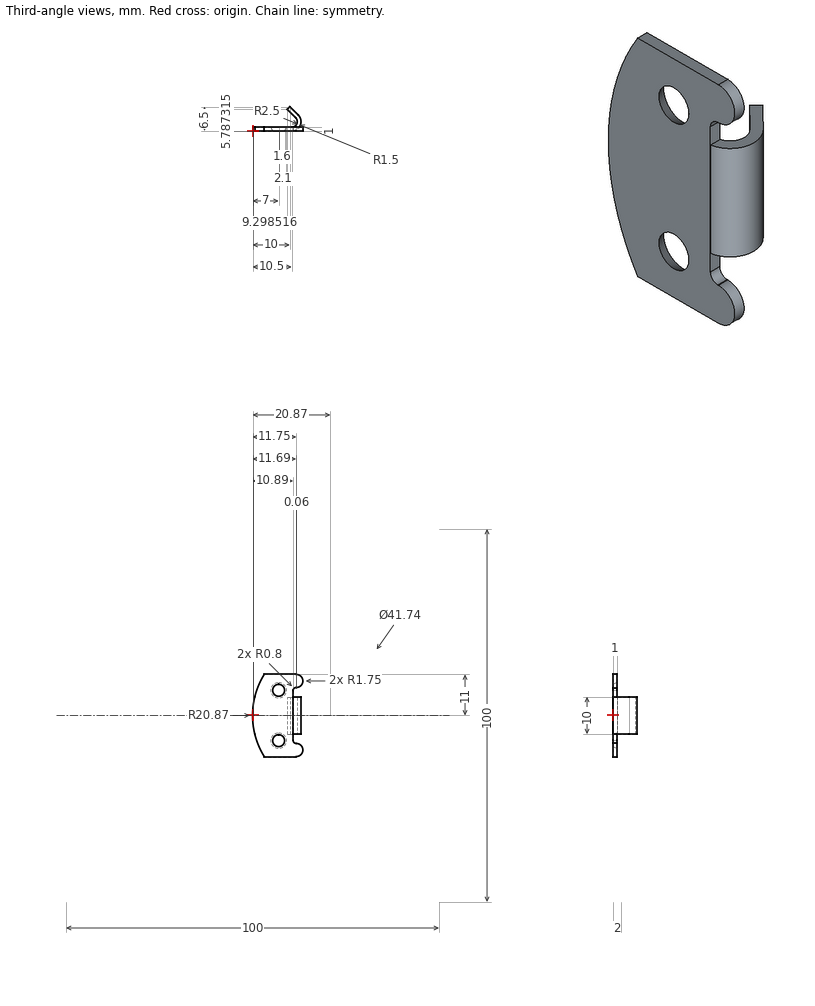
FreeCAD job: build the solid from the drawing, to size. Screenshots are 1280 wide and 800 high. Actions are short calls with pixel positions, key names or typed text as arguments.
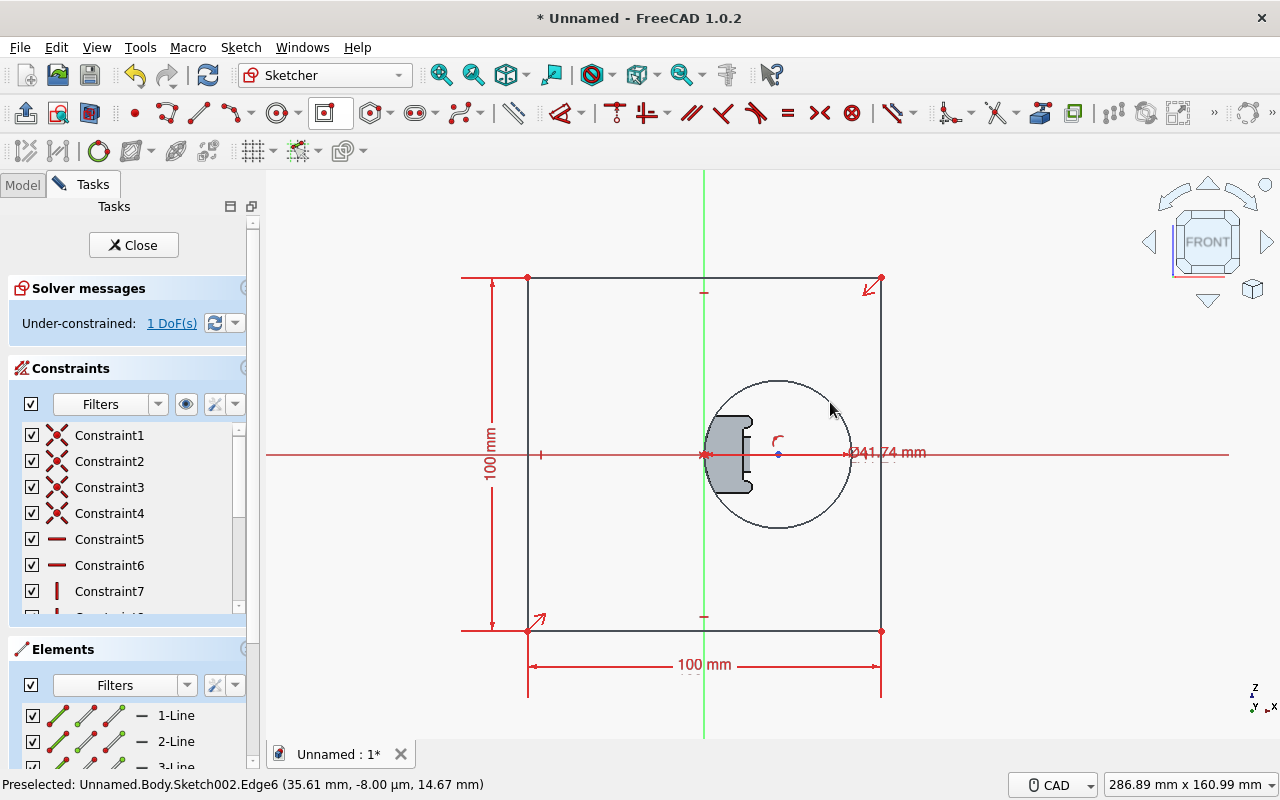
click(560, 114)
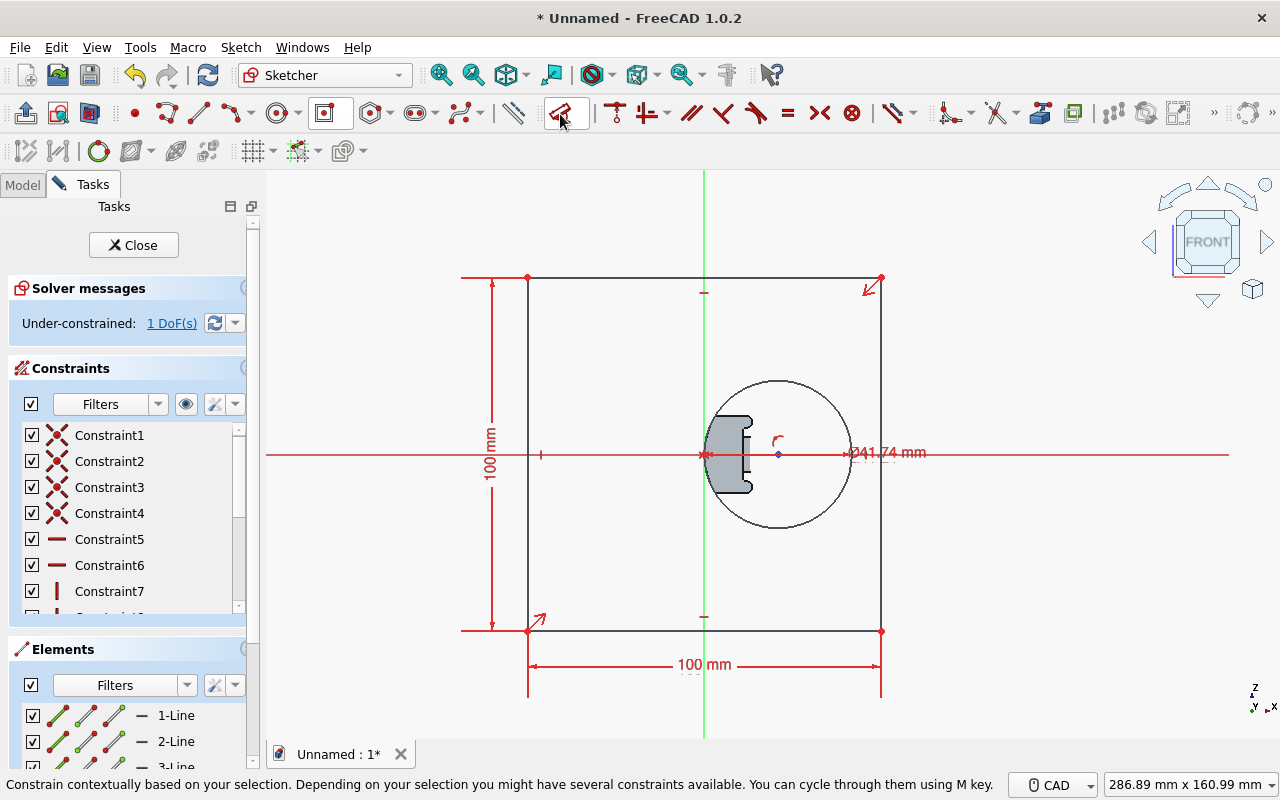
click(778, 455)
click(741, 489)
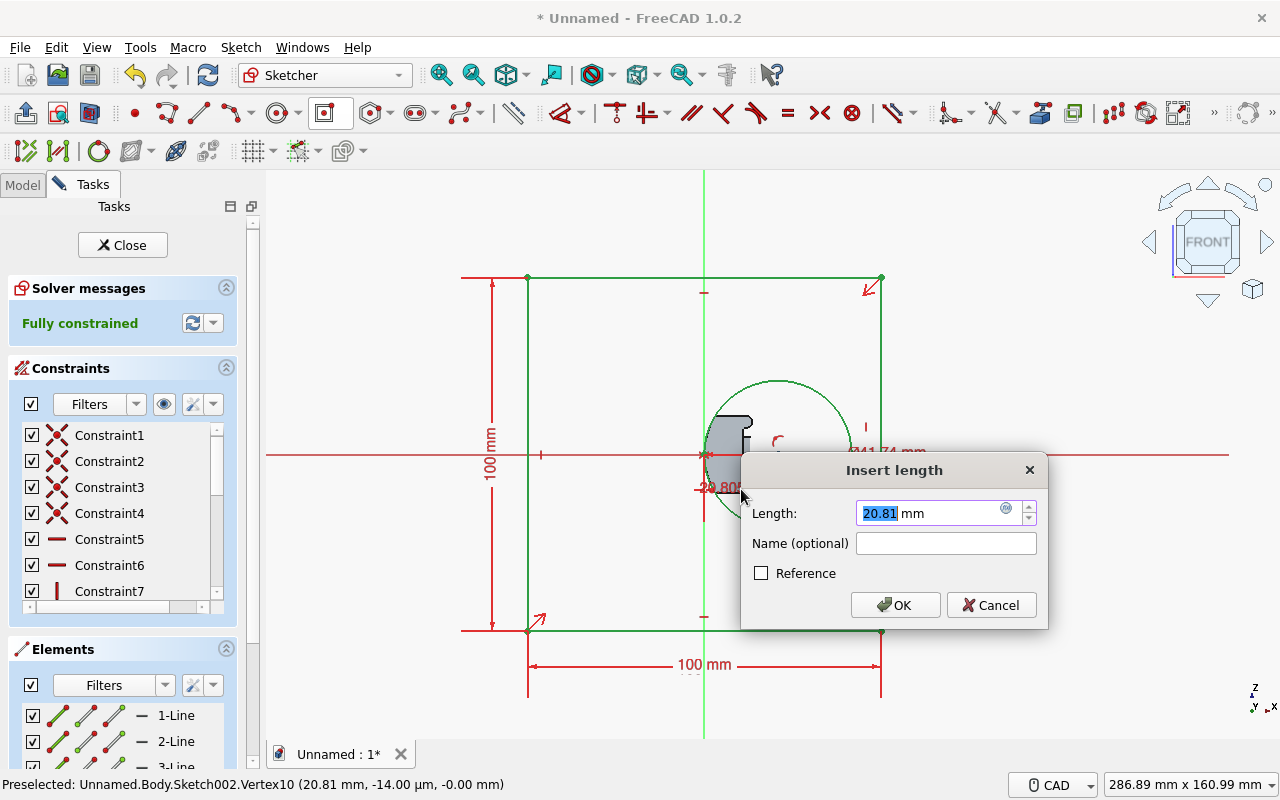
text(20.87)
key(Return)
key(Escape)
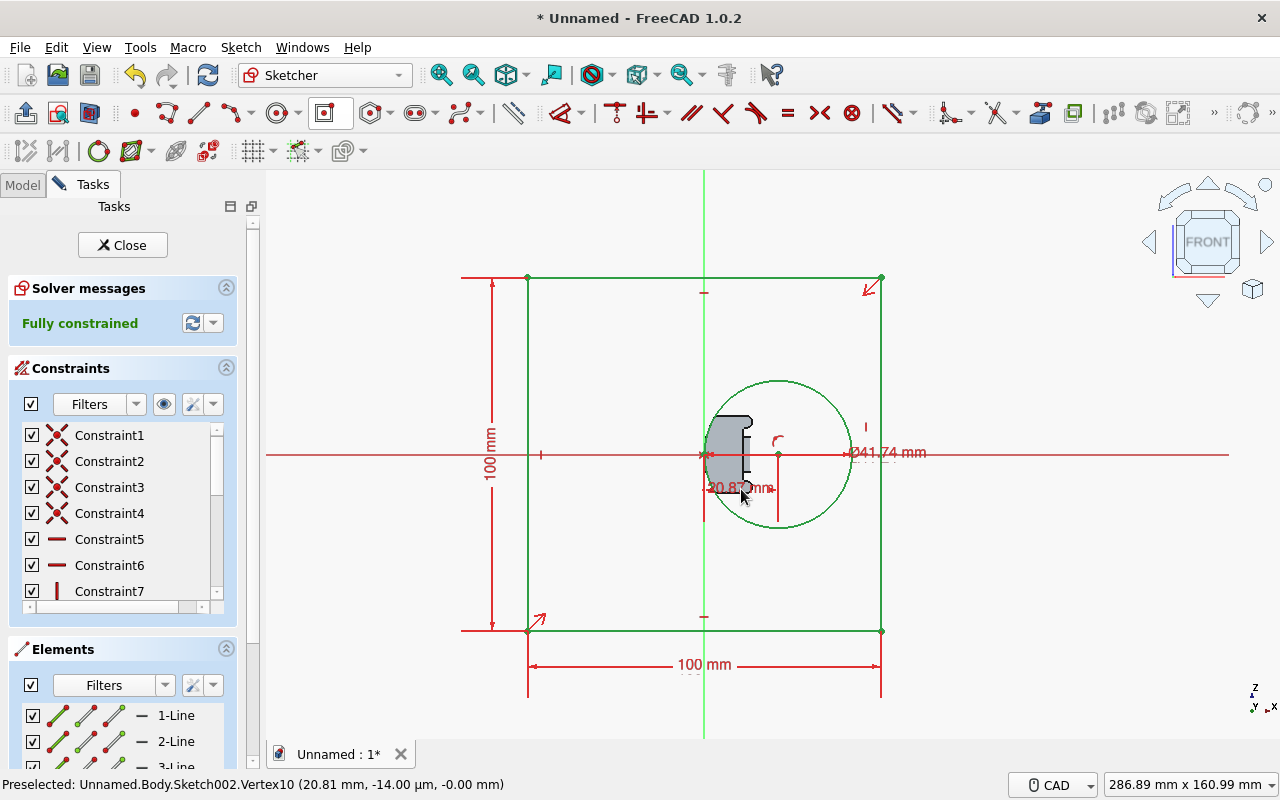
click(123, 245)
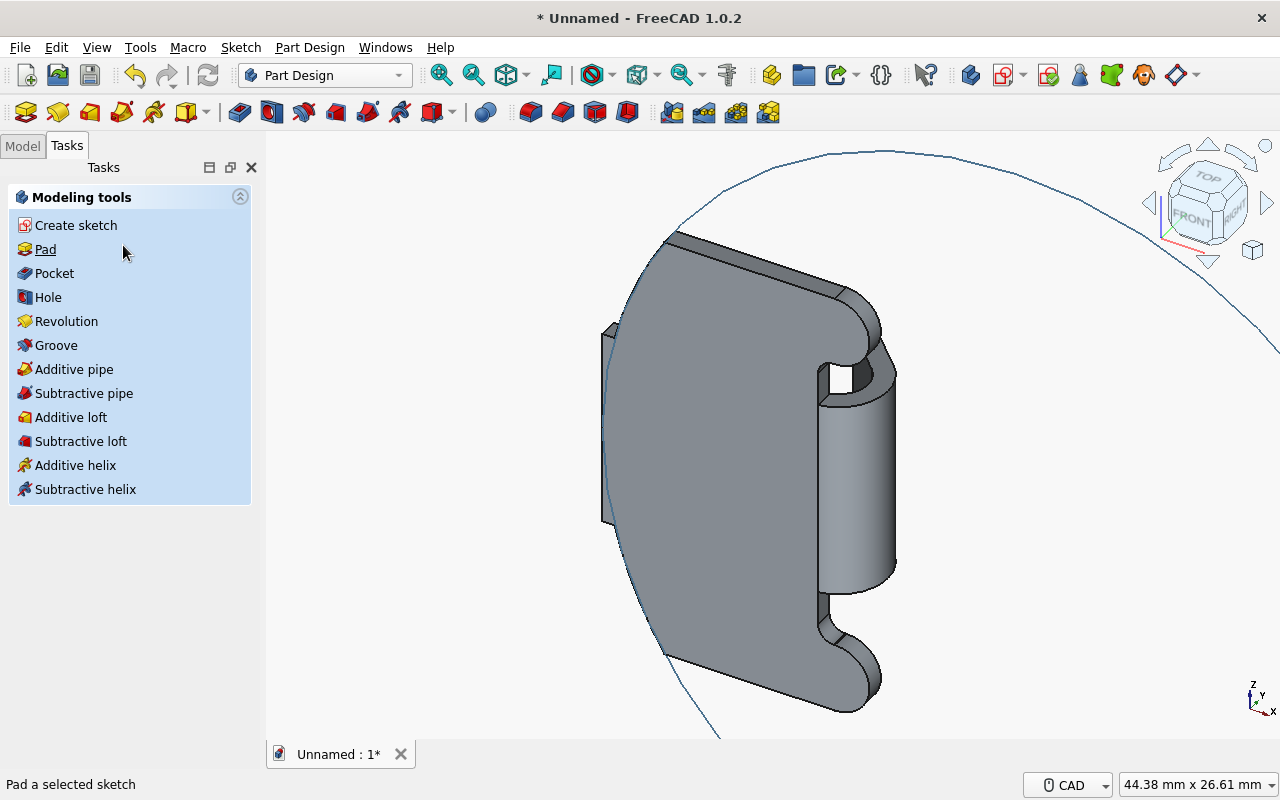
click(240, 112)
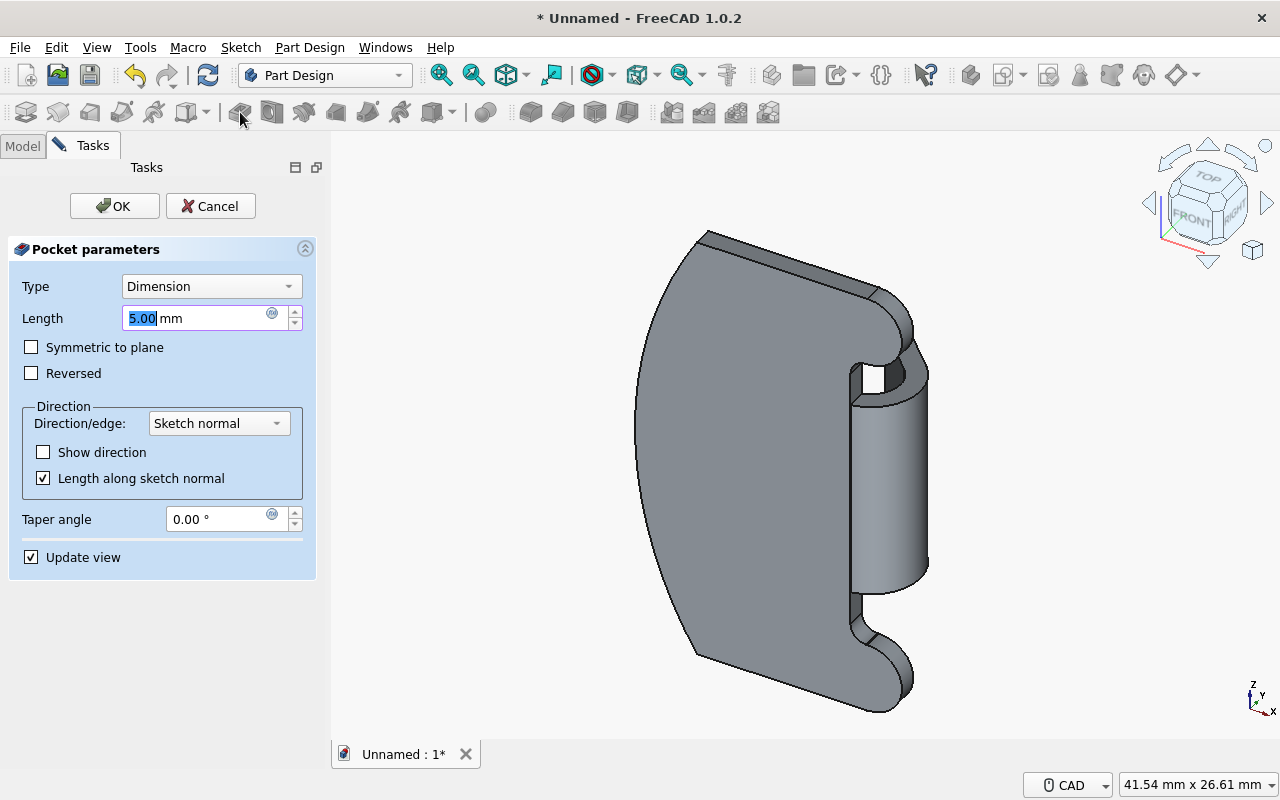
text(2)
key(Tab)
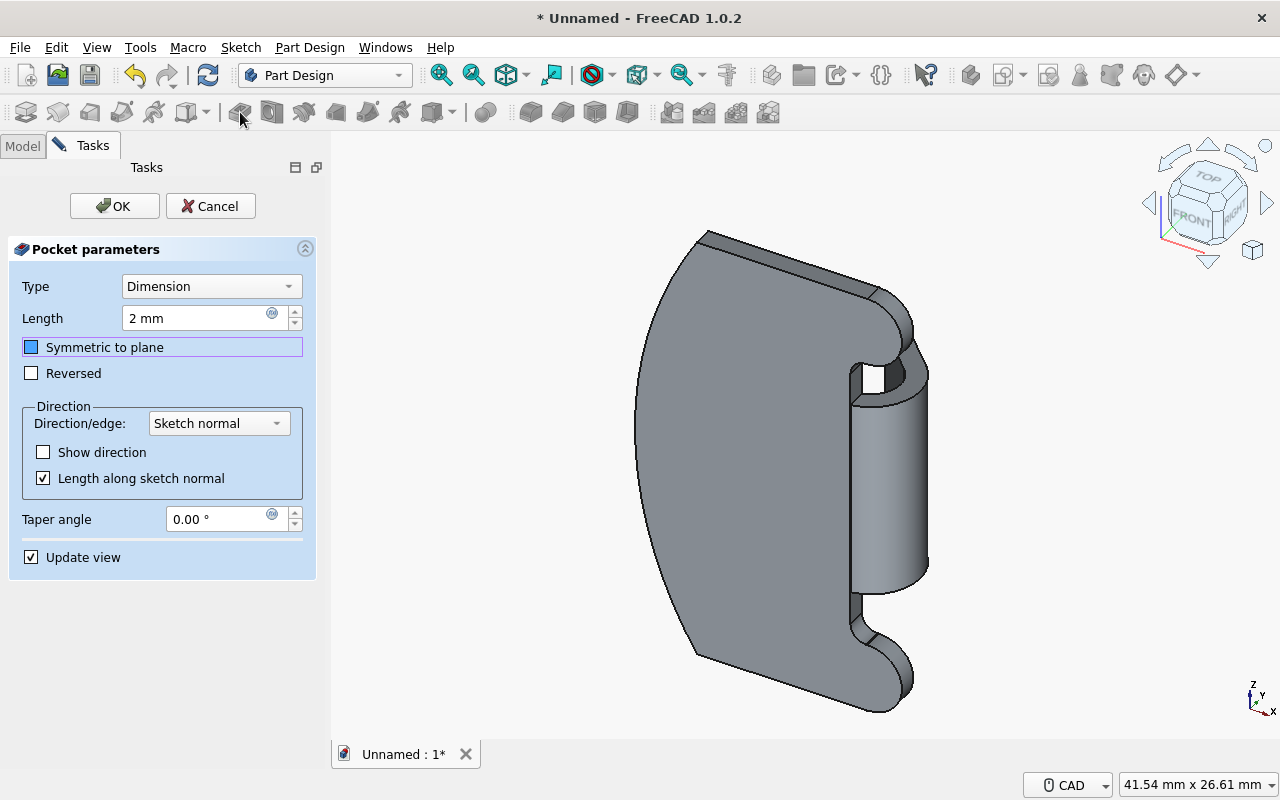
click(115, 206)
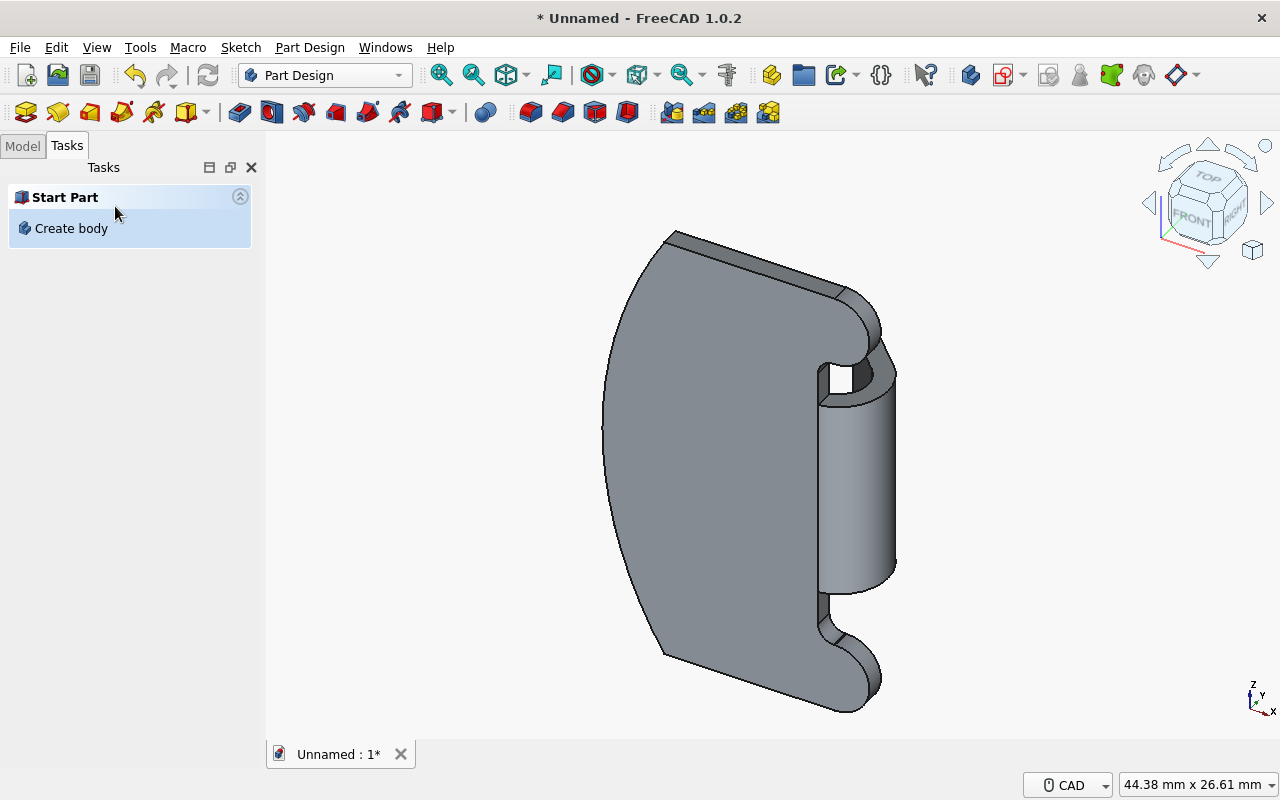
click(23, 145)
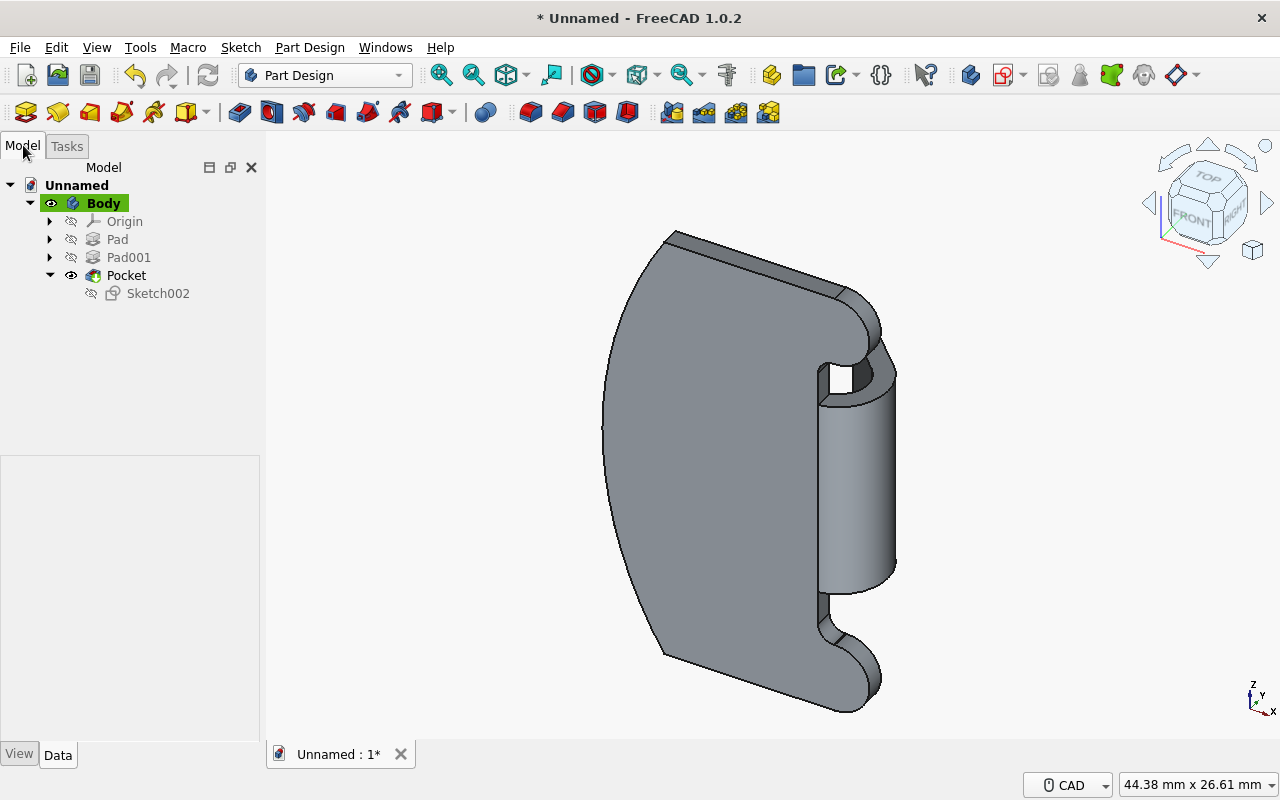
click(50, 221)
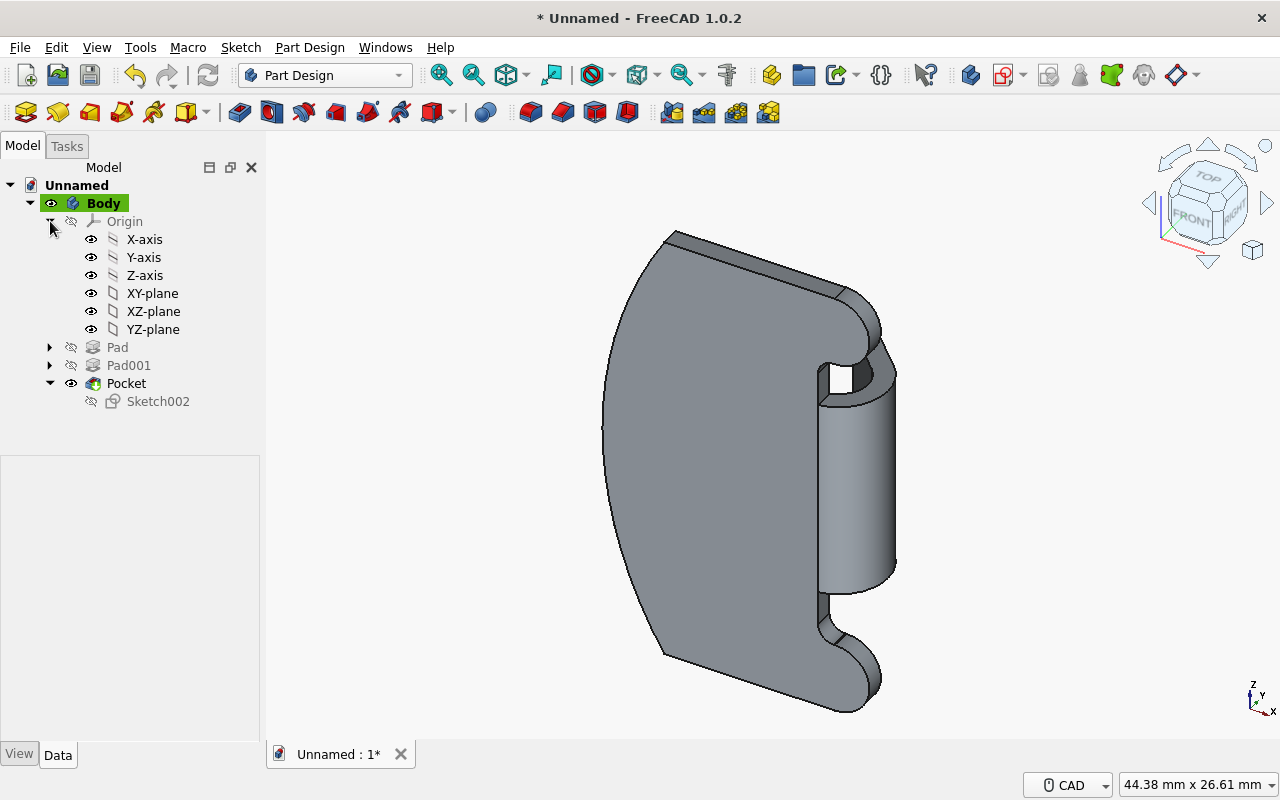
click(136, 293)